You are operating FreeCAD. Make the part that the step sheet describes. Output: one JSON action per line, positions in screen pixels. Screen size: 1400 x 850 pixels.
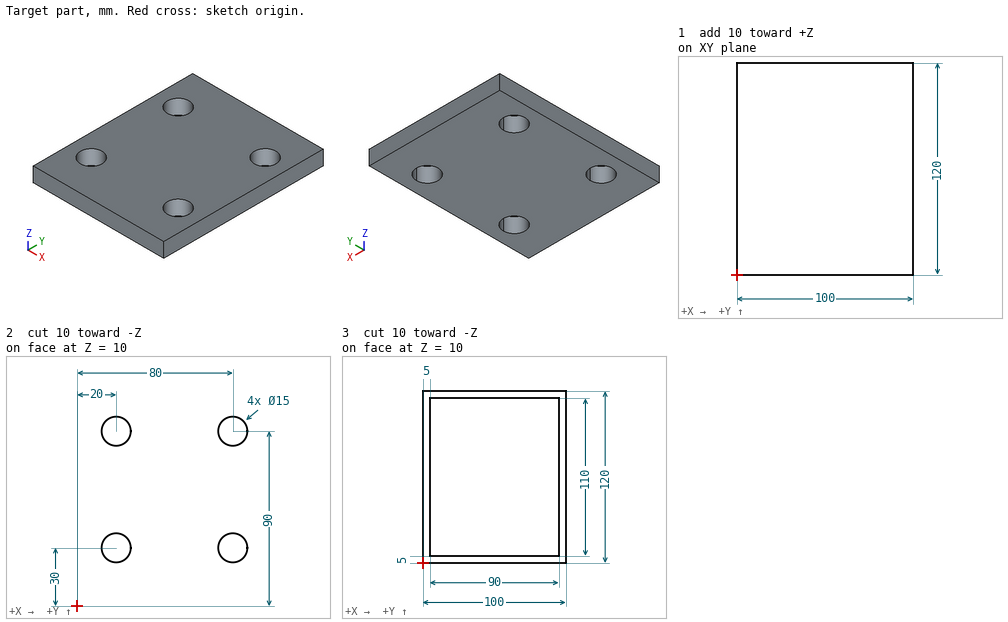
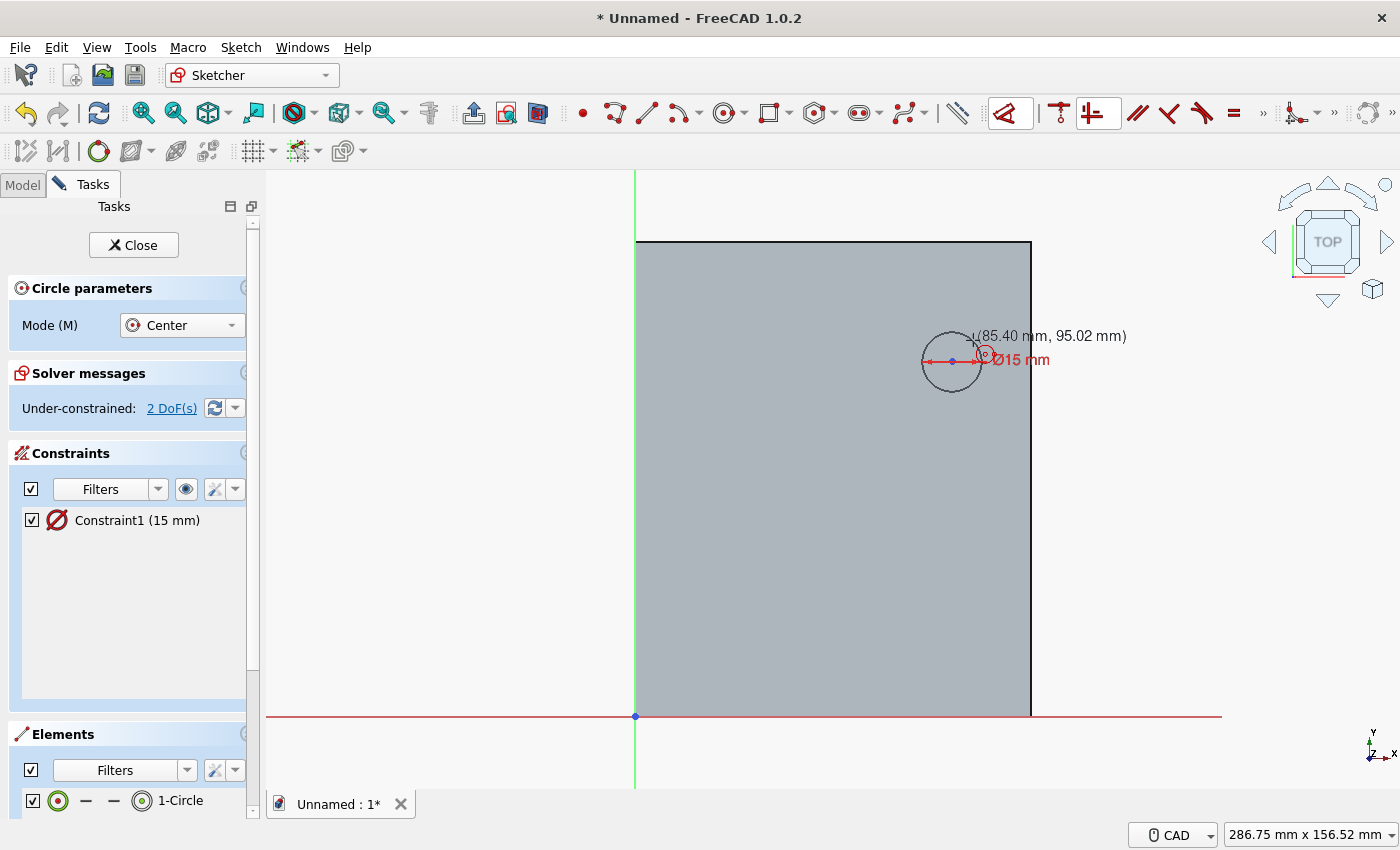
{"action": "left_click", "coordinate": [714, 361]}
{"action": "mouse_move", "coordinate": [735, 340]}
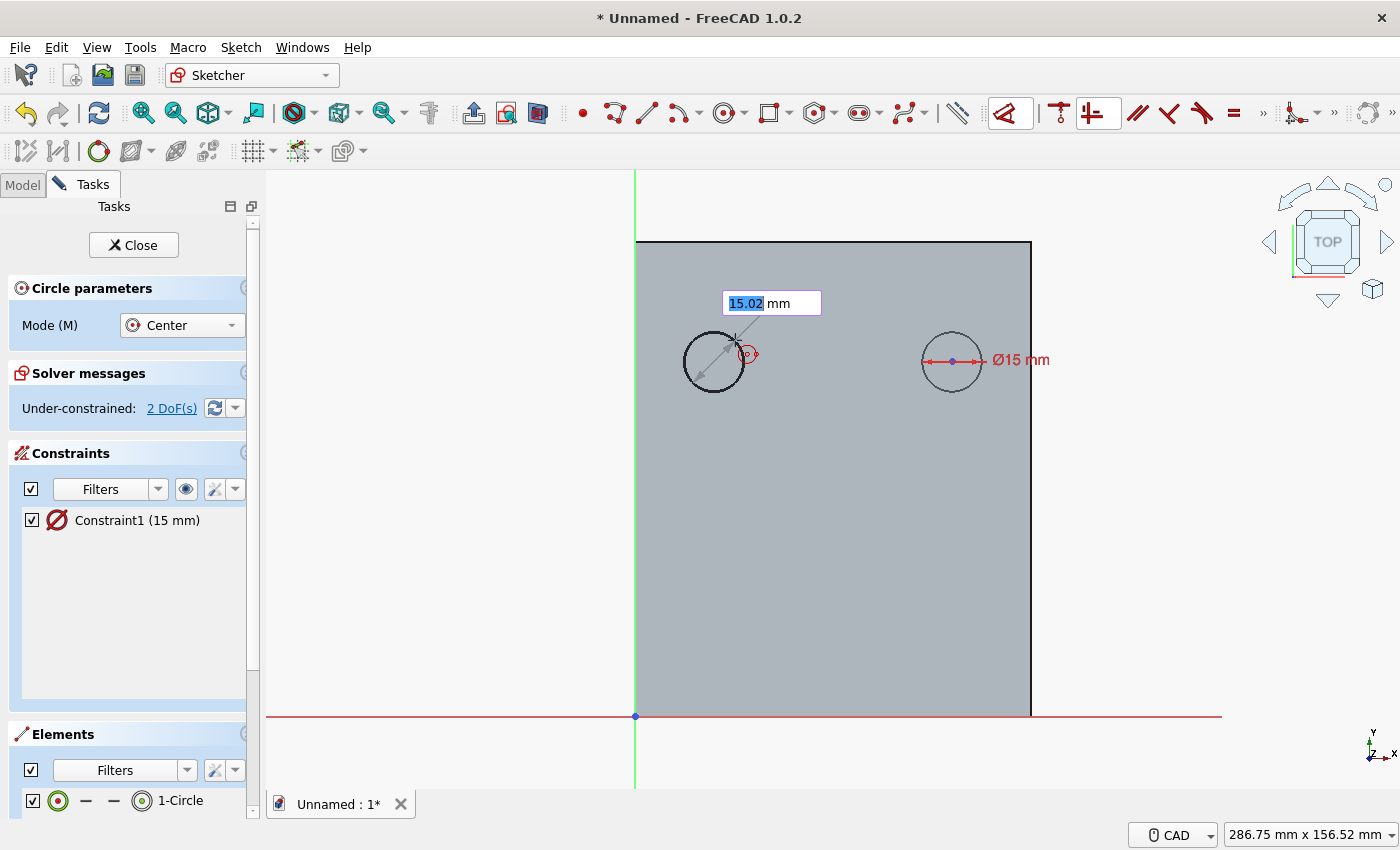
{"action": "type", "text": "15"}
{"action": "key", "text": "Return"}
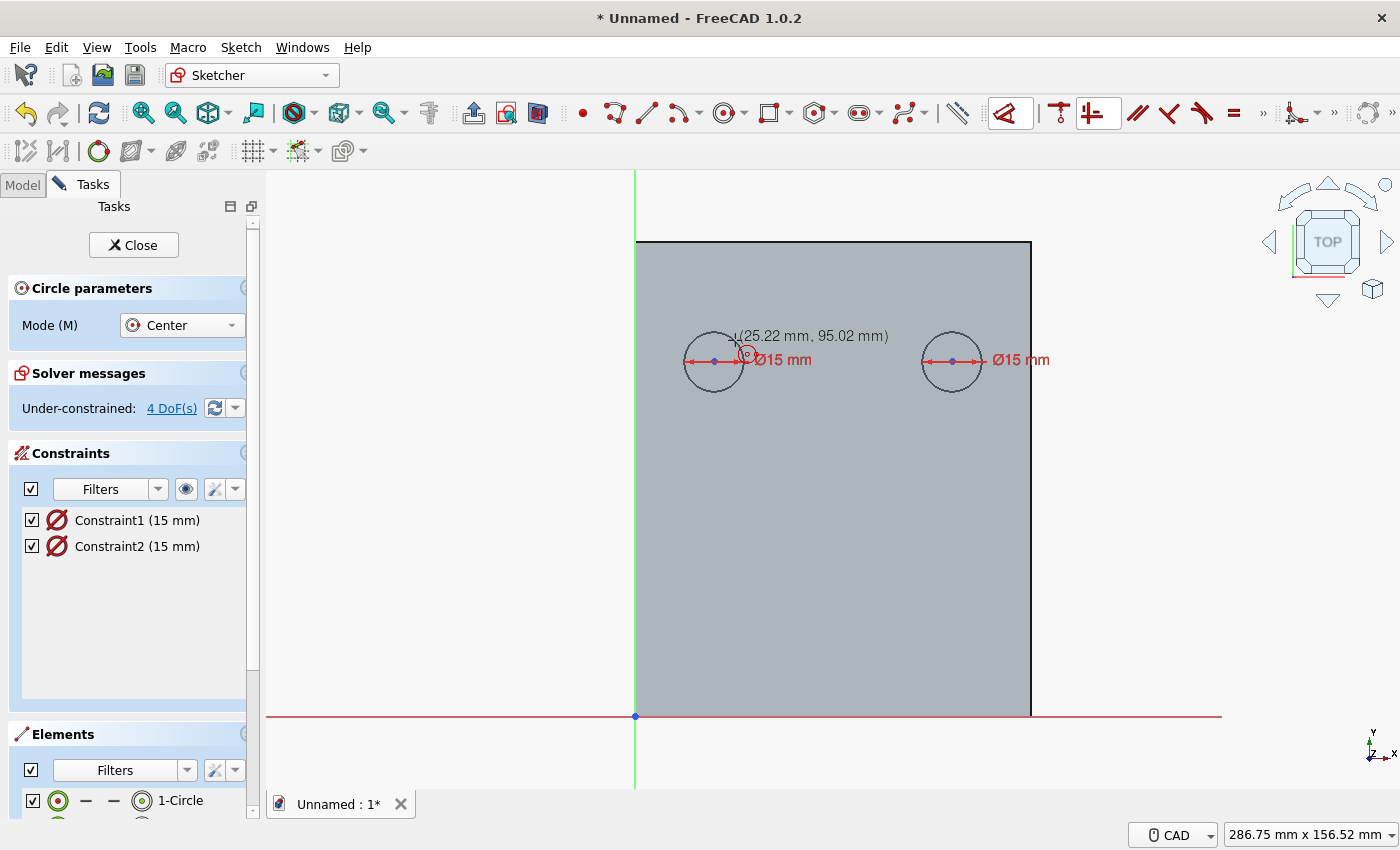
{"action": "left_click", "coordinate": [714, 598]}
{"action": "mouse_move", "coordinate": [735, 577]}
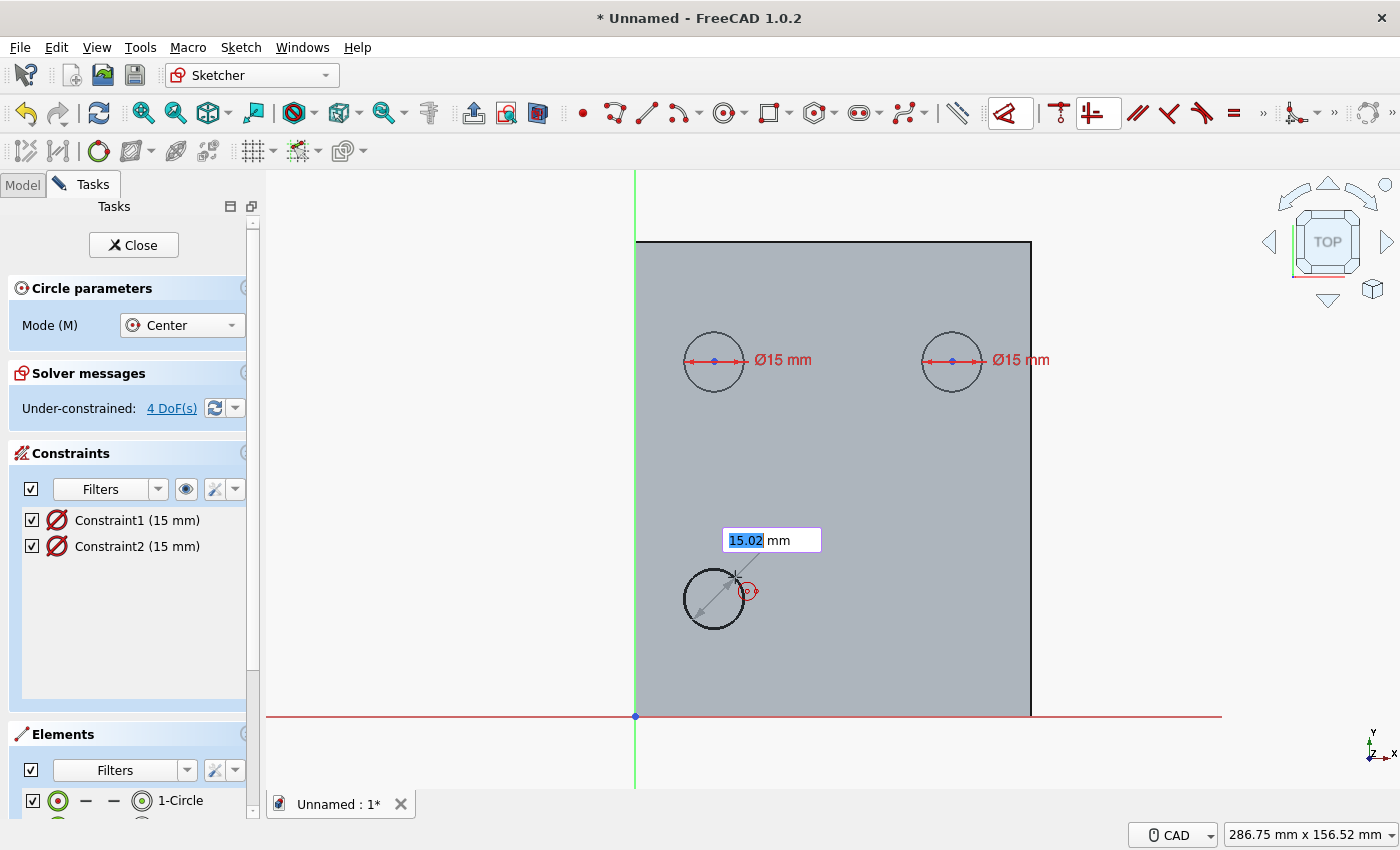
{"action": "type", "text": "15"}
{"action": "key", "text": "Return"}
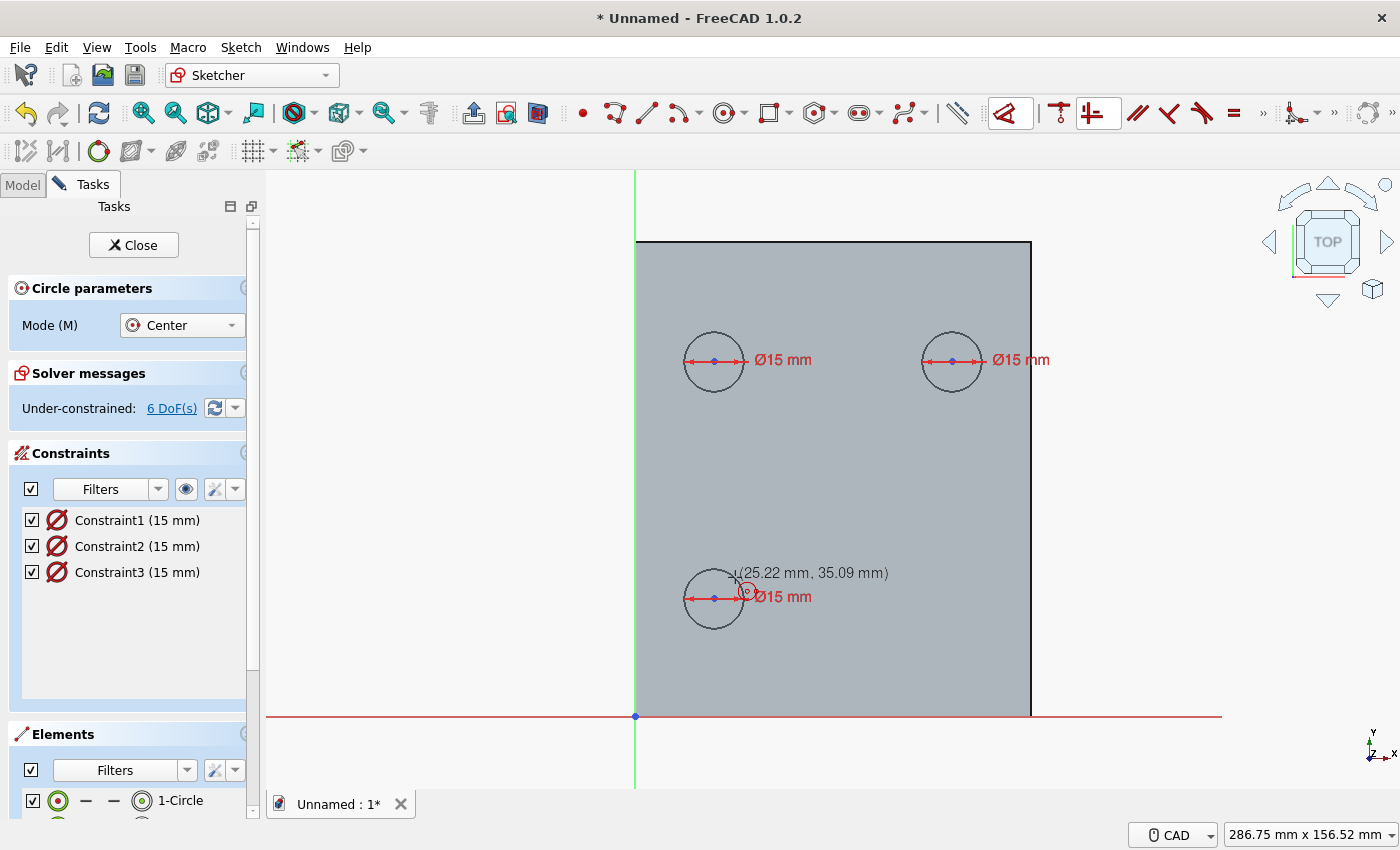
{"action": "left_click", "coordinate": [952, 598]}
{"action": "mouse_move", "coordinate": [973, 577]}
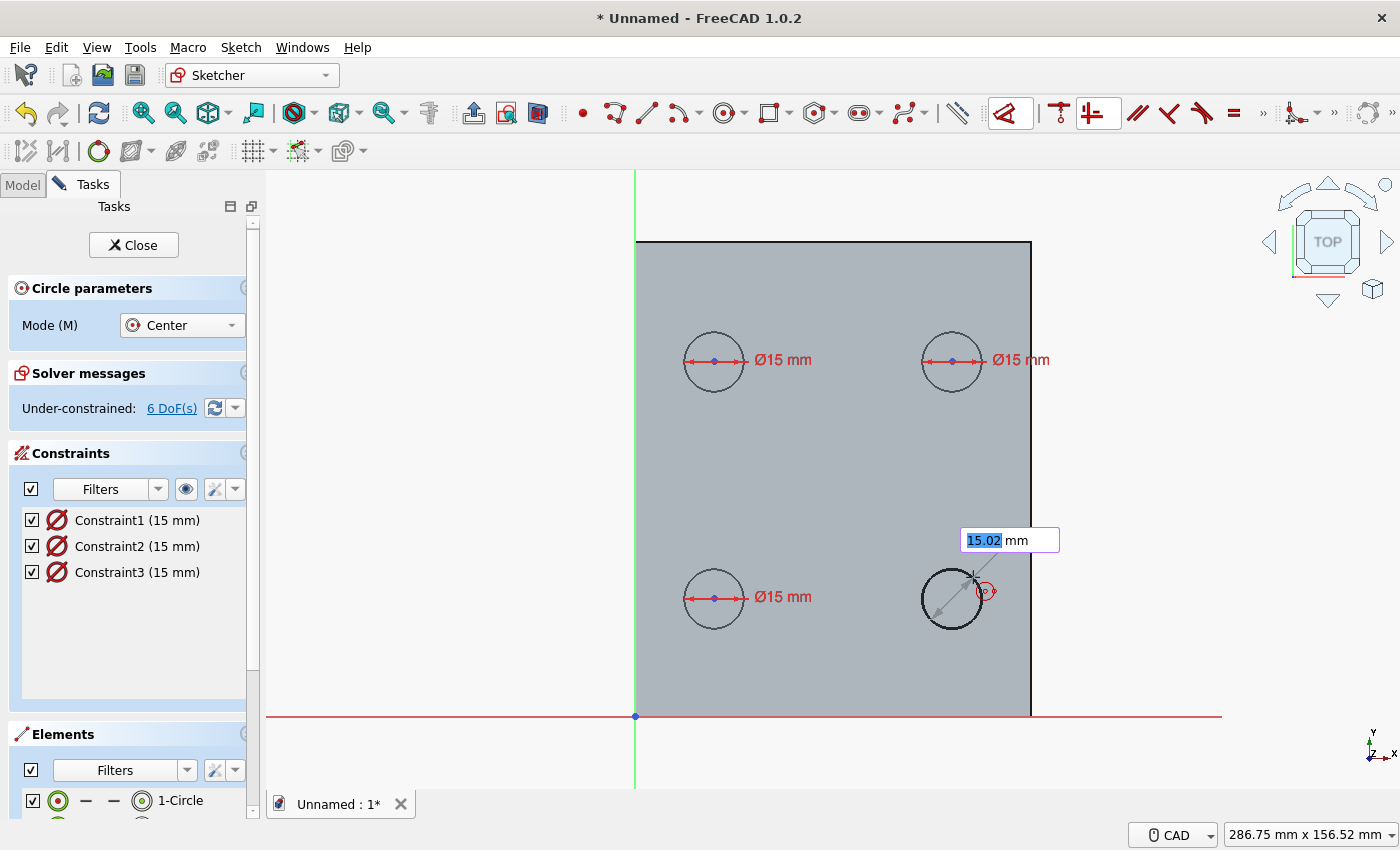
{"action": "type", "text": "15"}
{"action": "key", "text": "Return"}
{"action": "key", "text": "Escape"}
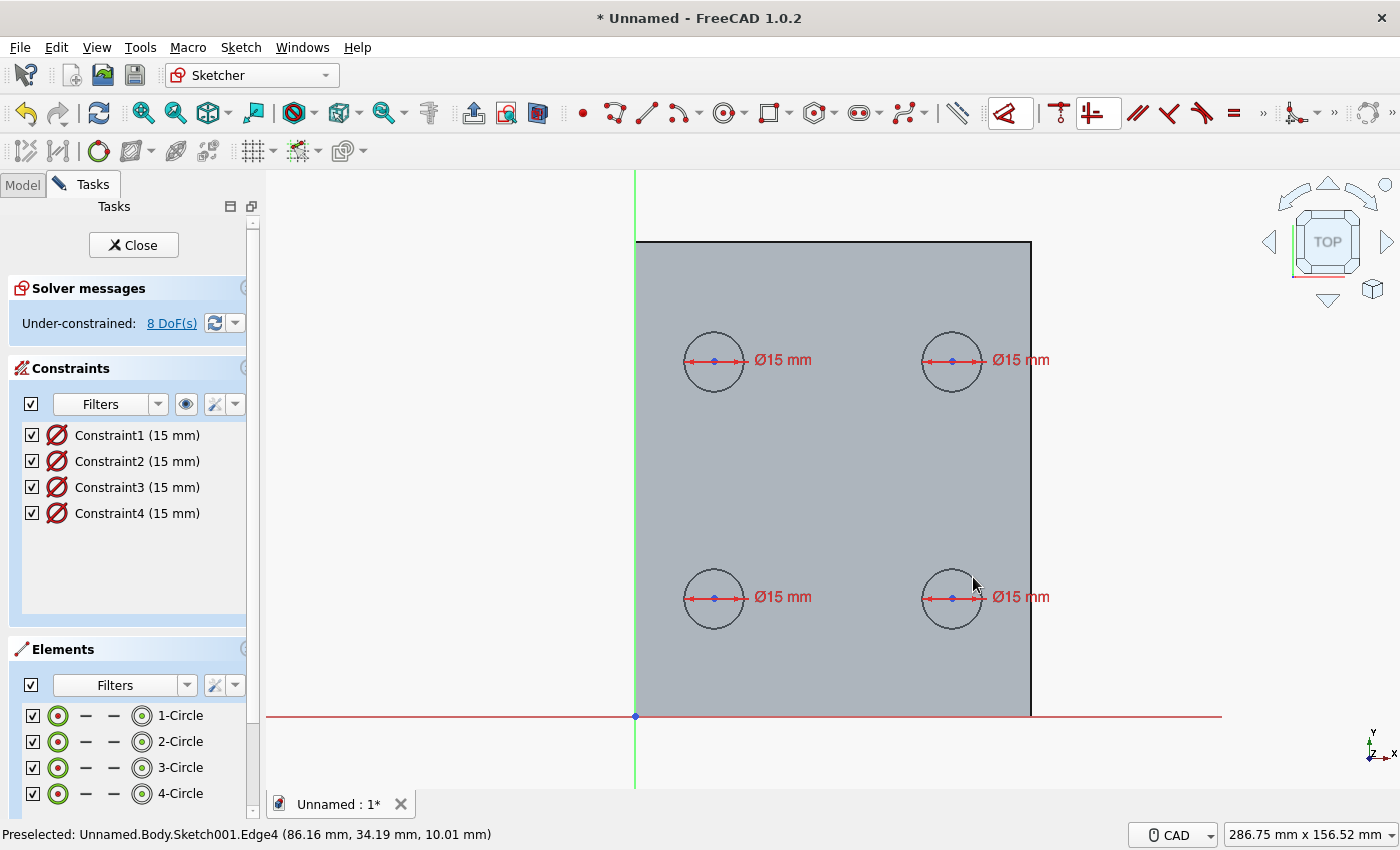
{"action": "left_click", "coordinate": [952, 362]}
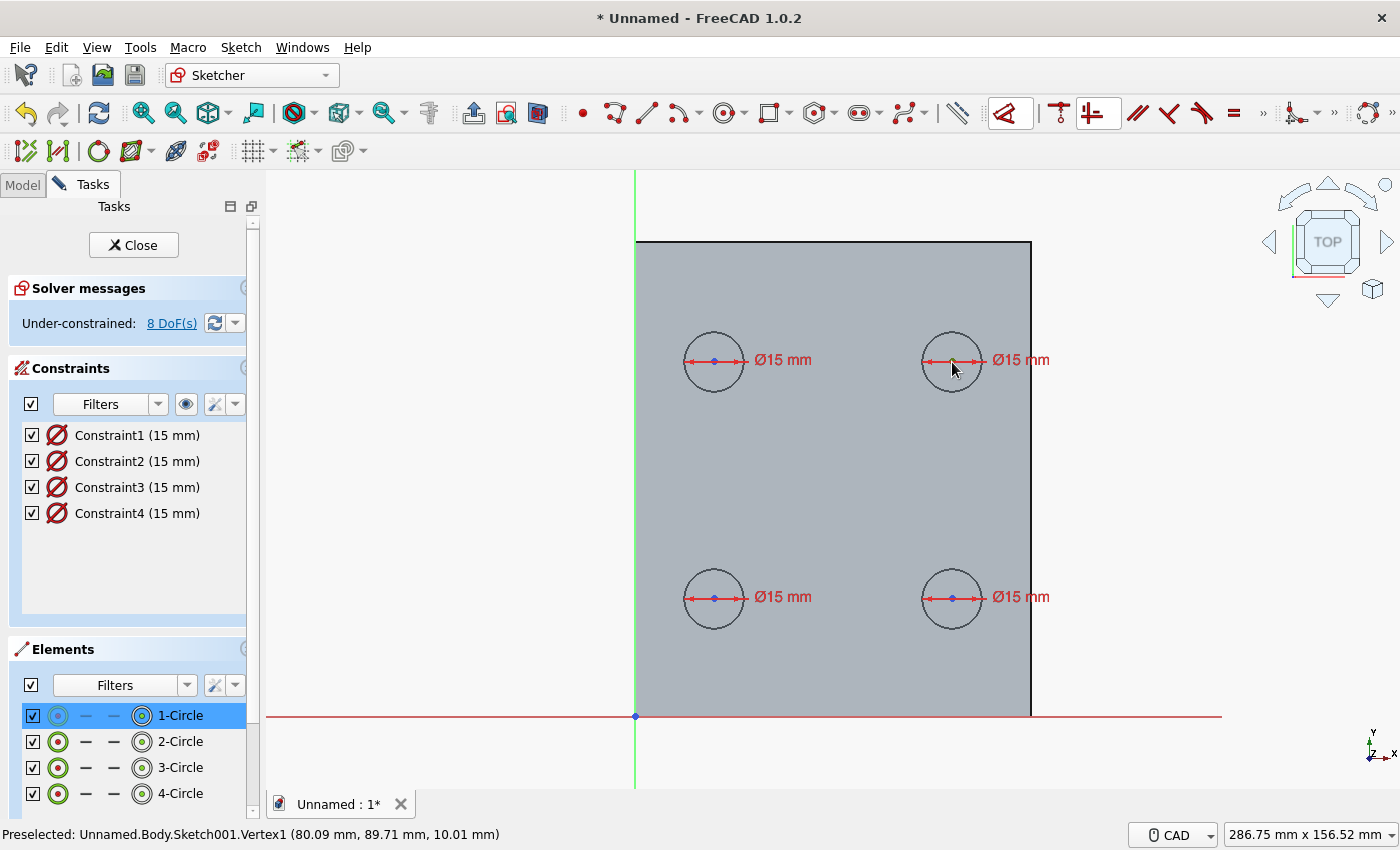
{"action": "left_click", "coordinate": [714, 362]}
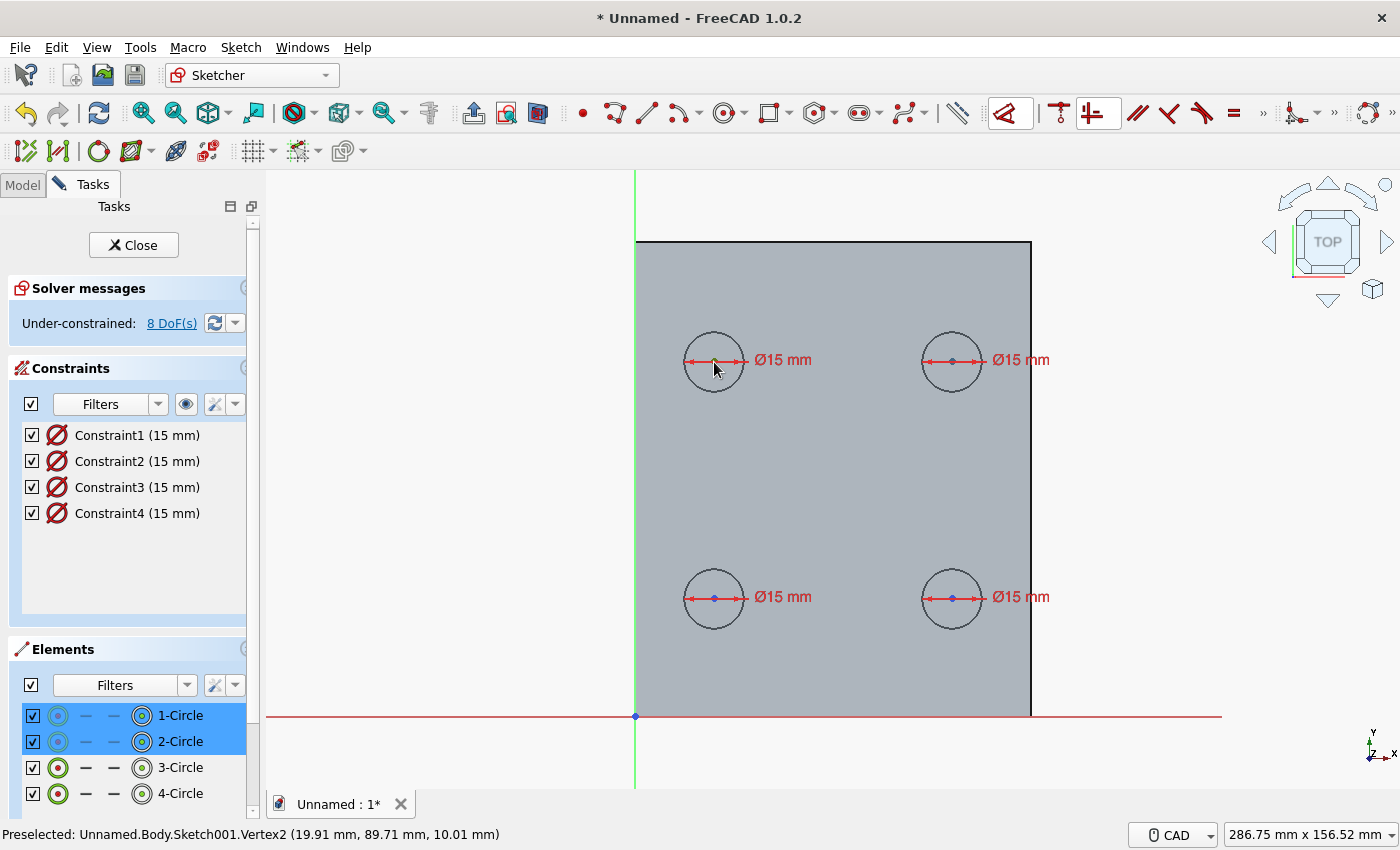
{"action": "key", "text": "h"}